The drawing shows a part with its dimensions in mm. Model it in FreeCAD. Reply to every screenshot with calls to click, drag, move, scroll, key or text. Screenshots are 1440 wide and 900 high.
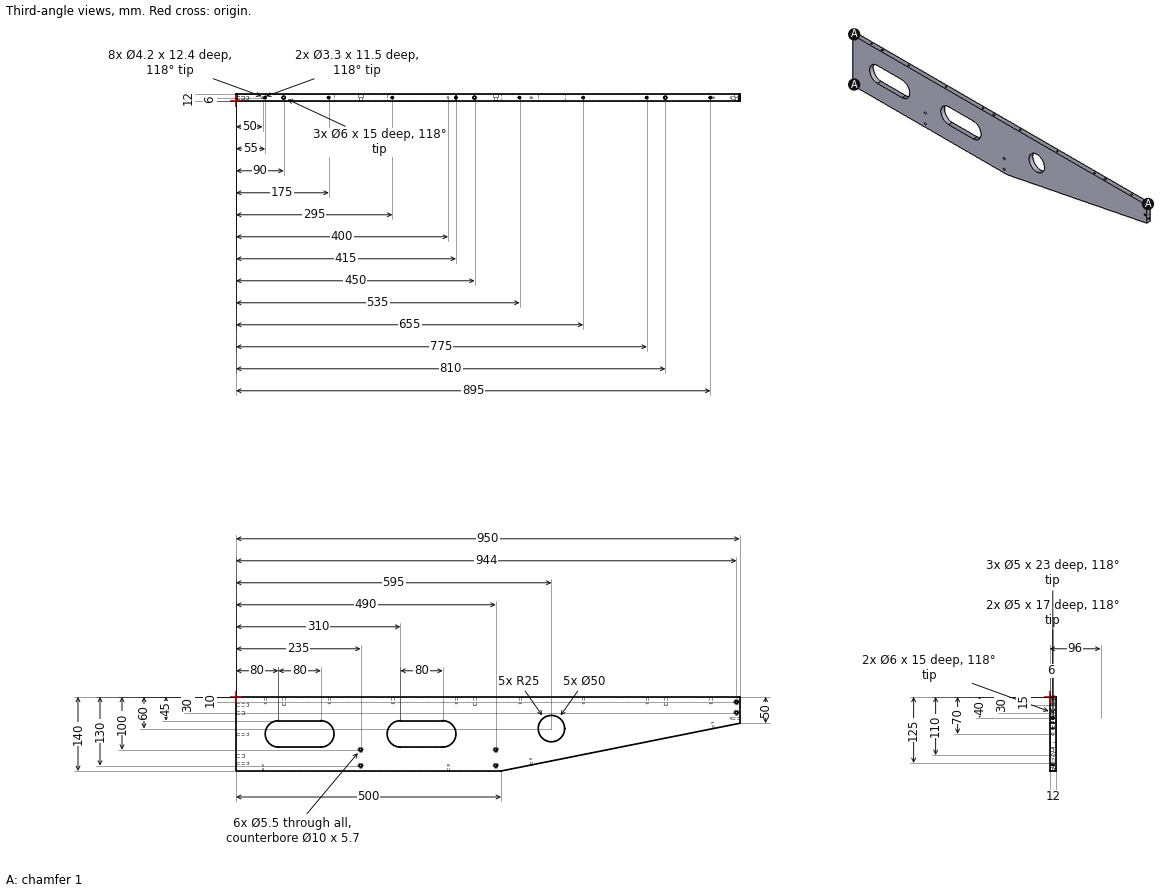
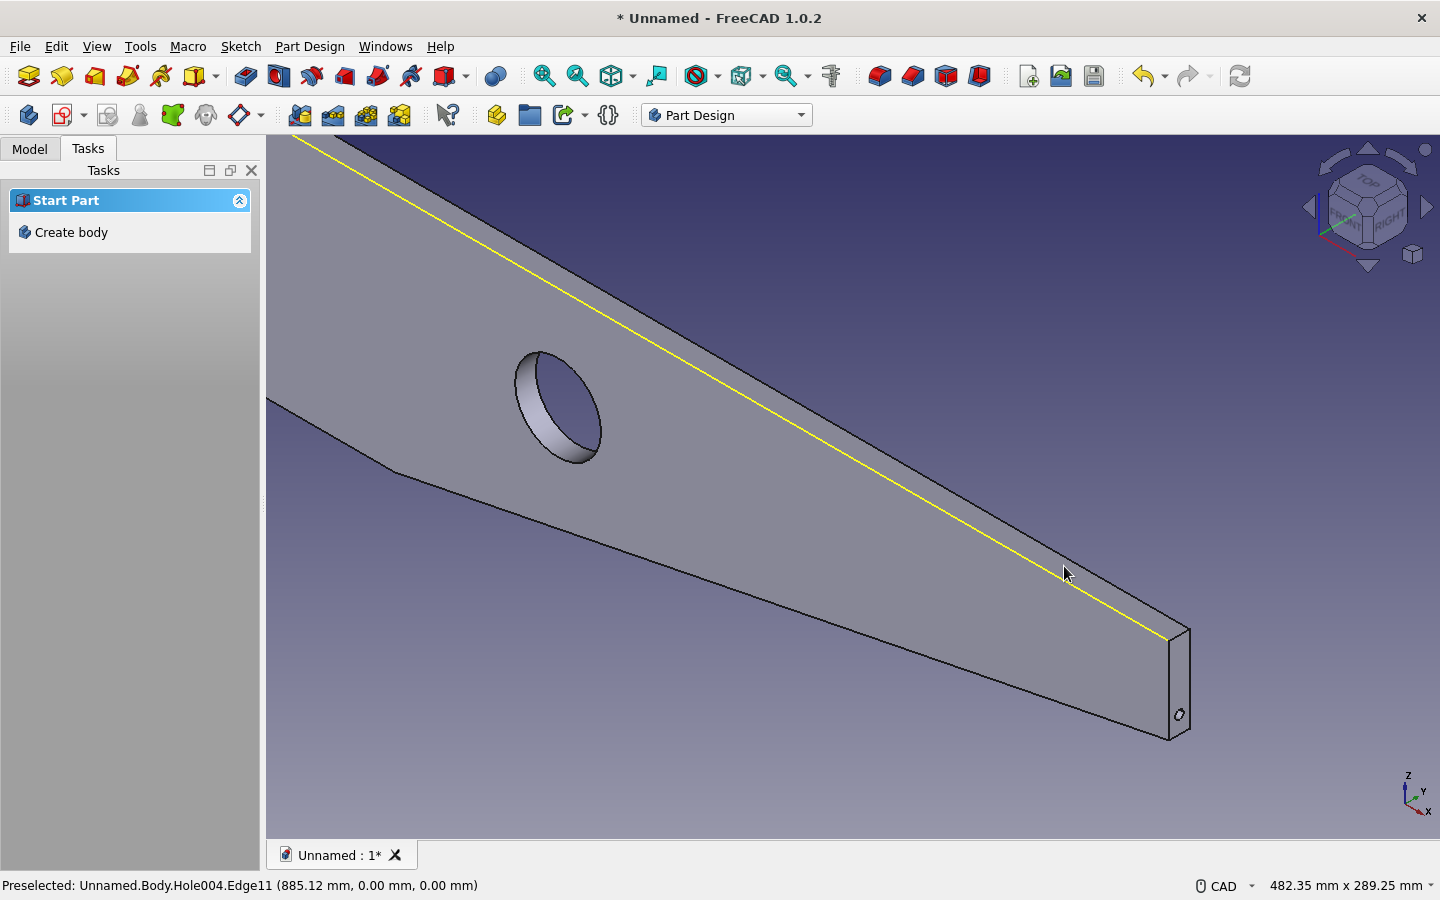
click(1063, 567)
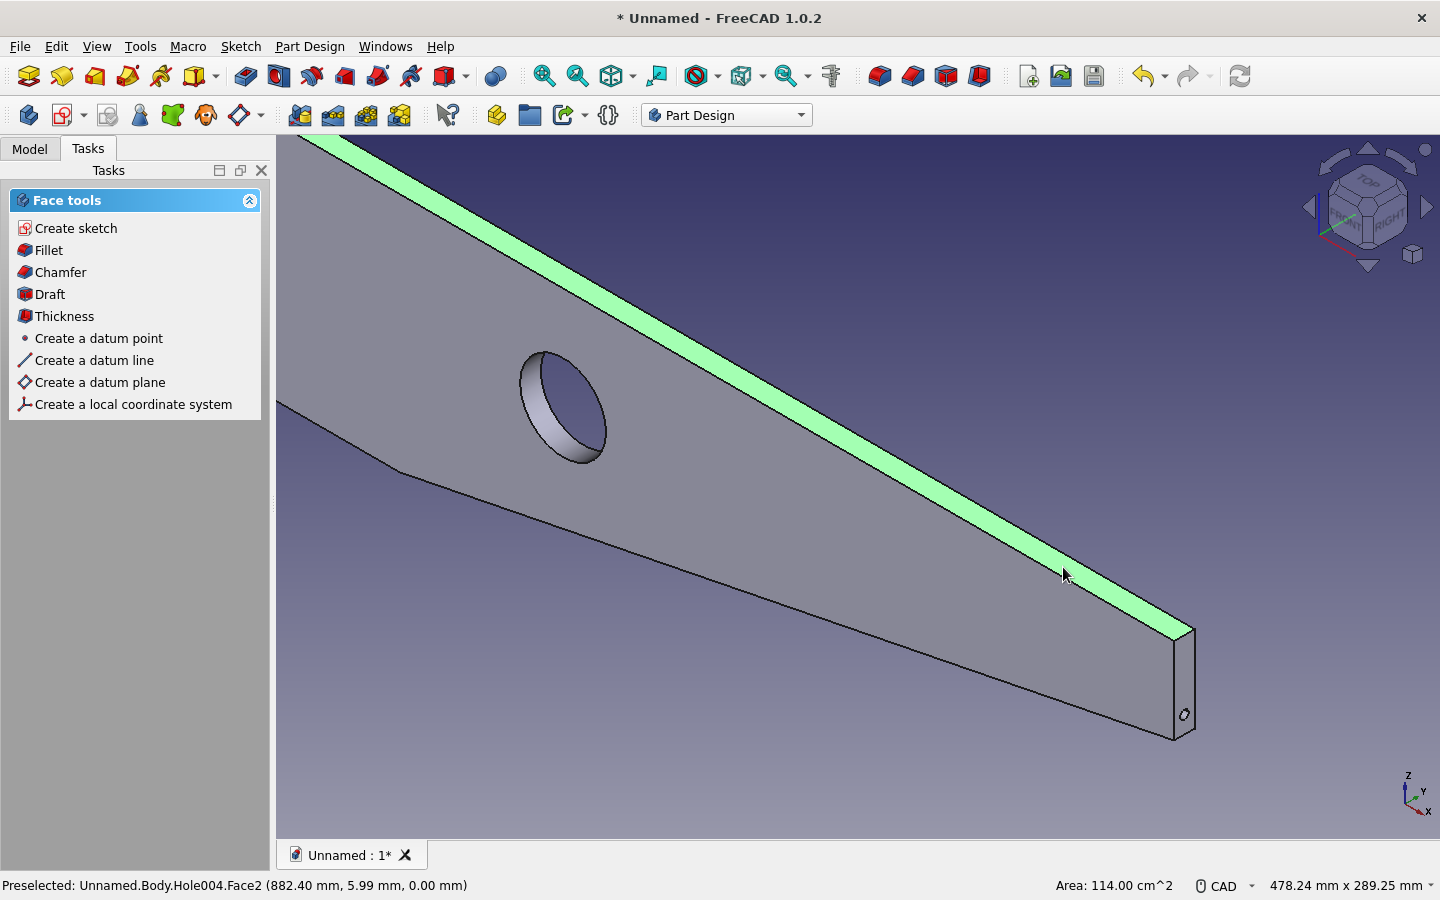
click(62, 116)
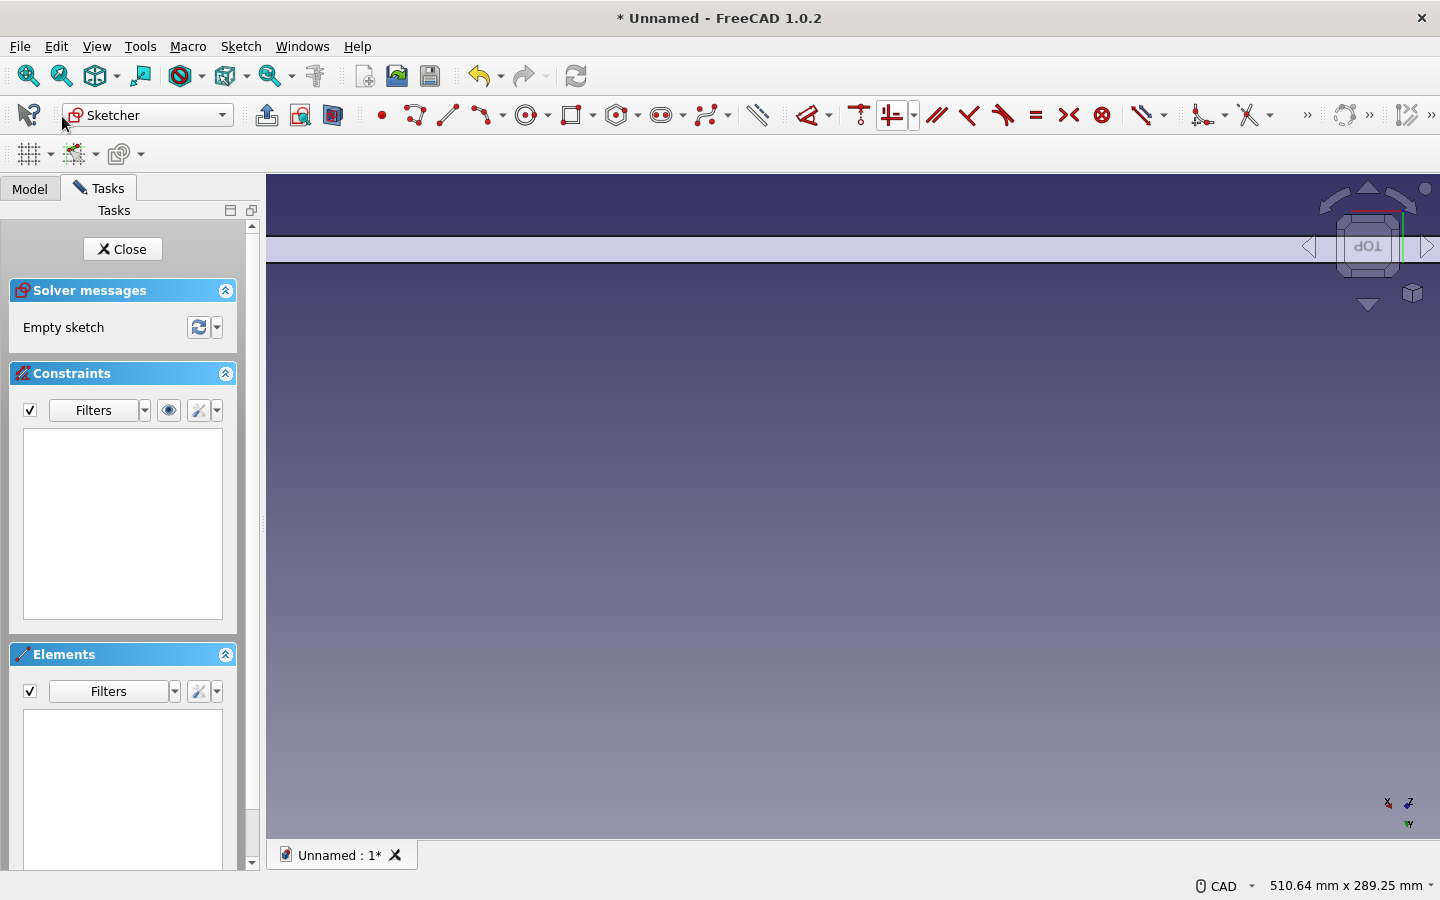
scroll(477, 659, down, 5)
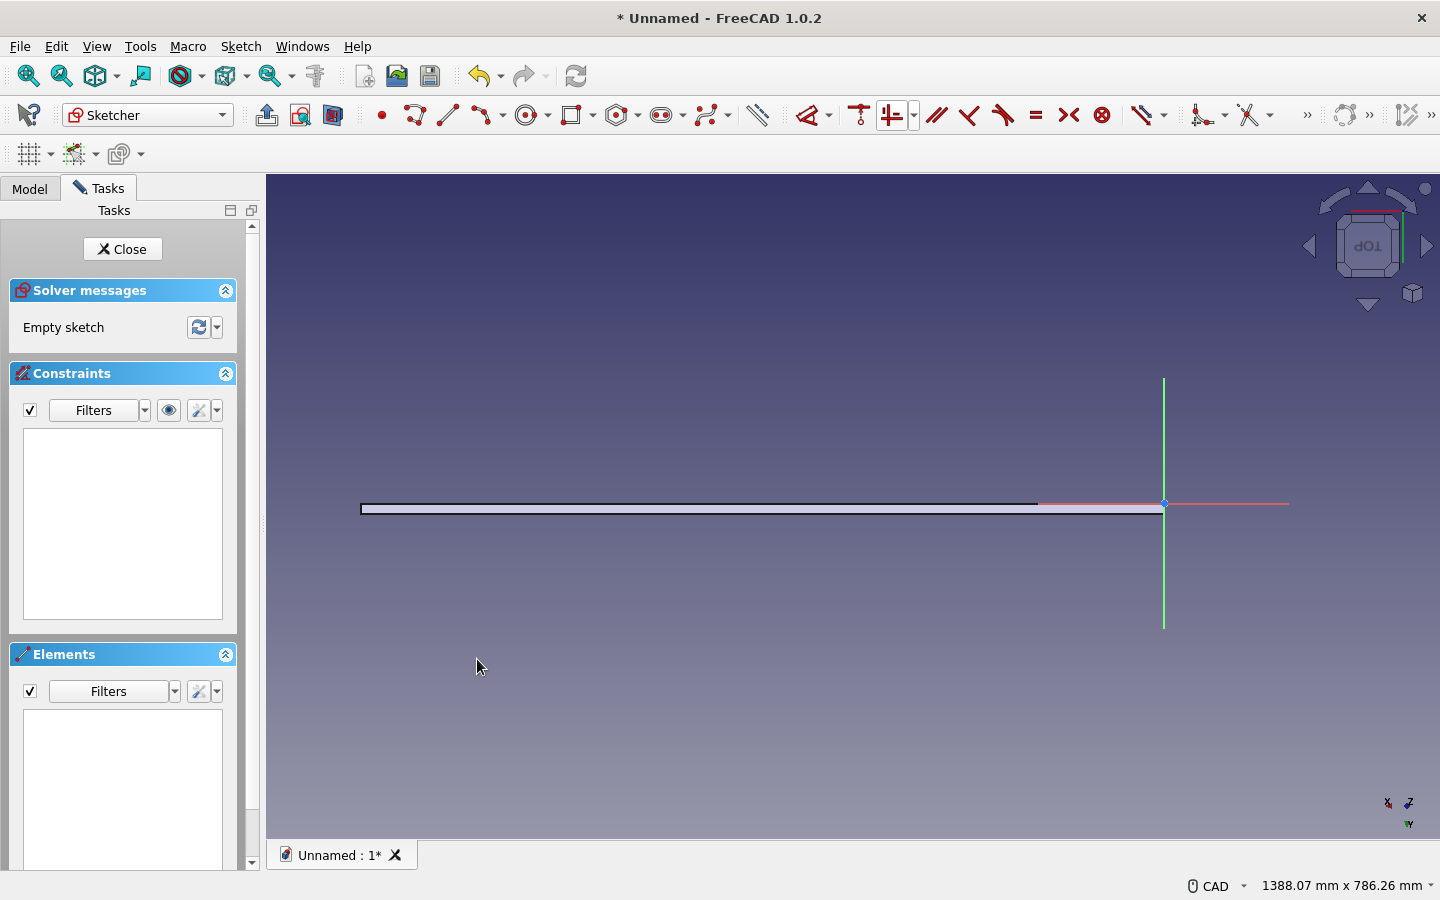
click(526, 116)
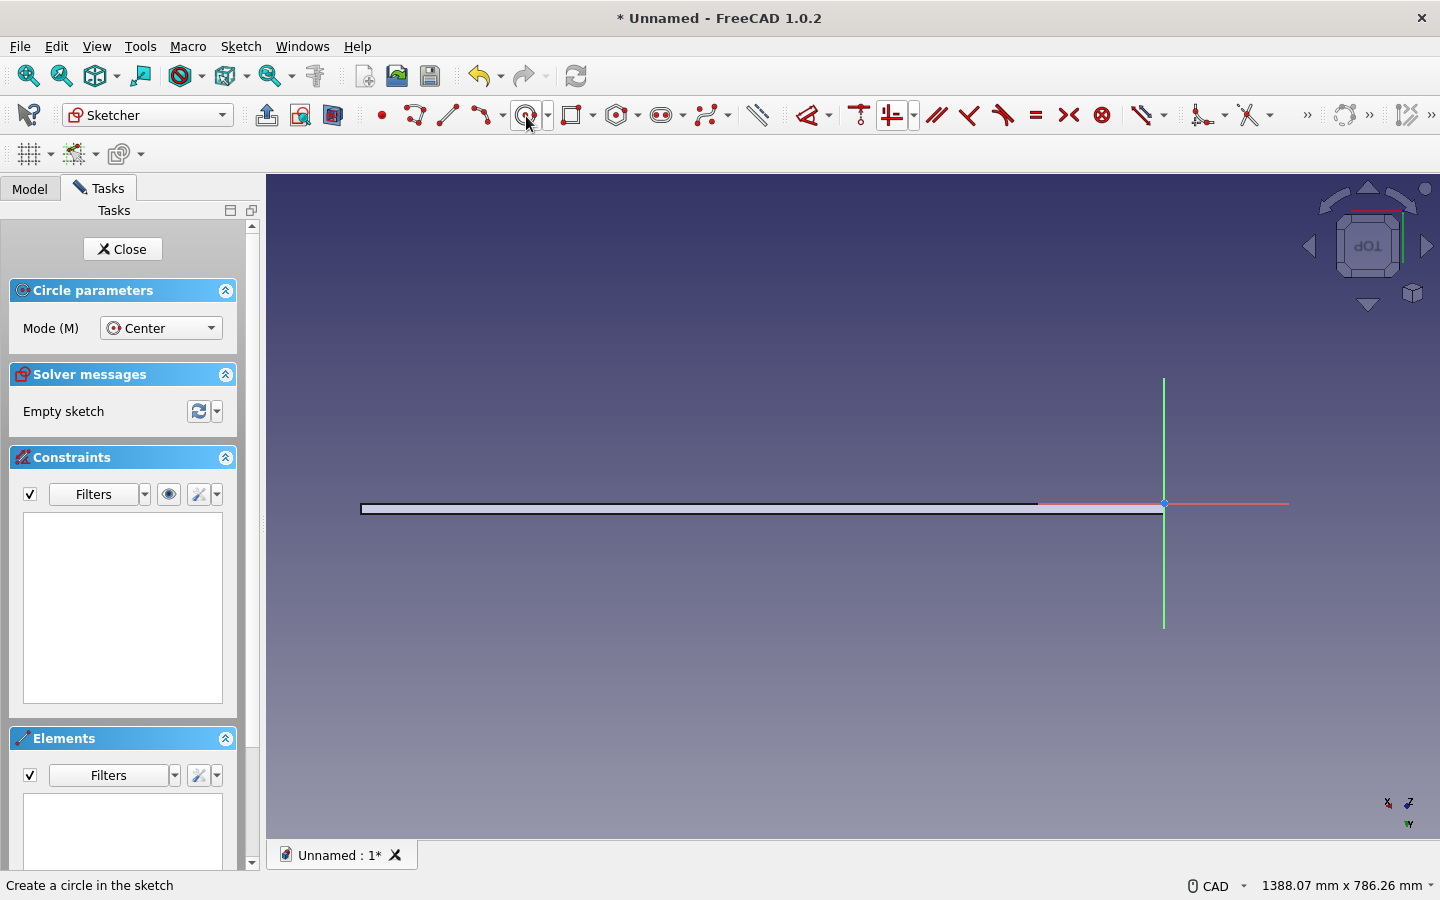
scroll(1118, 509, up, 13)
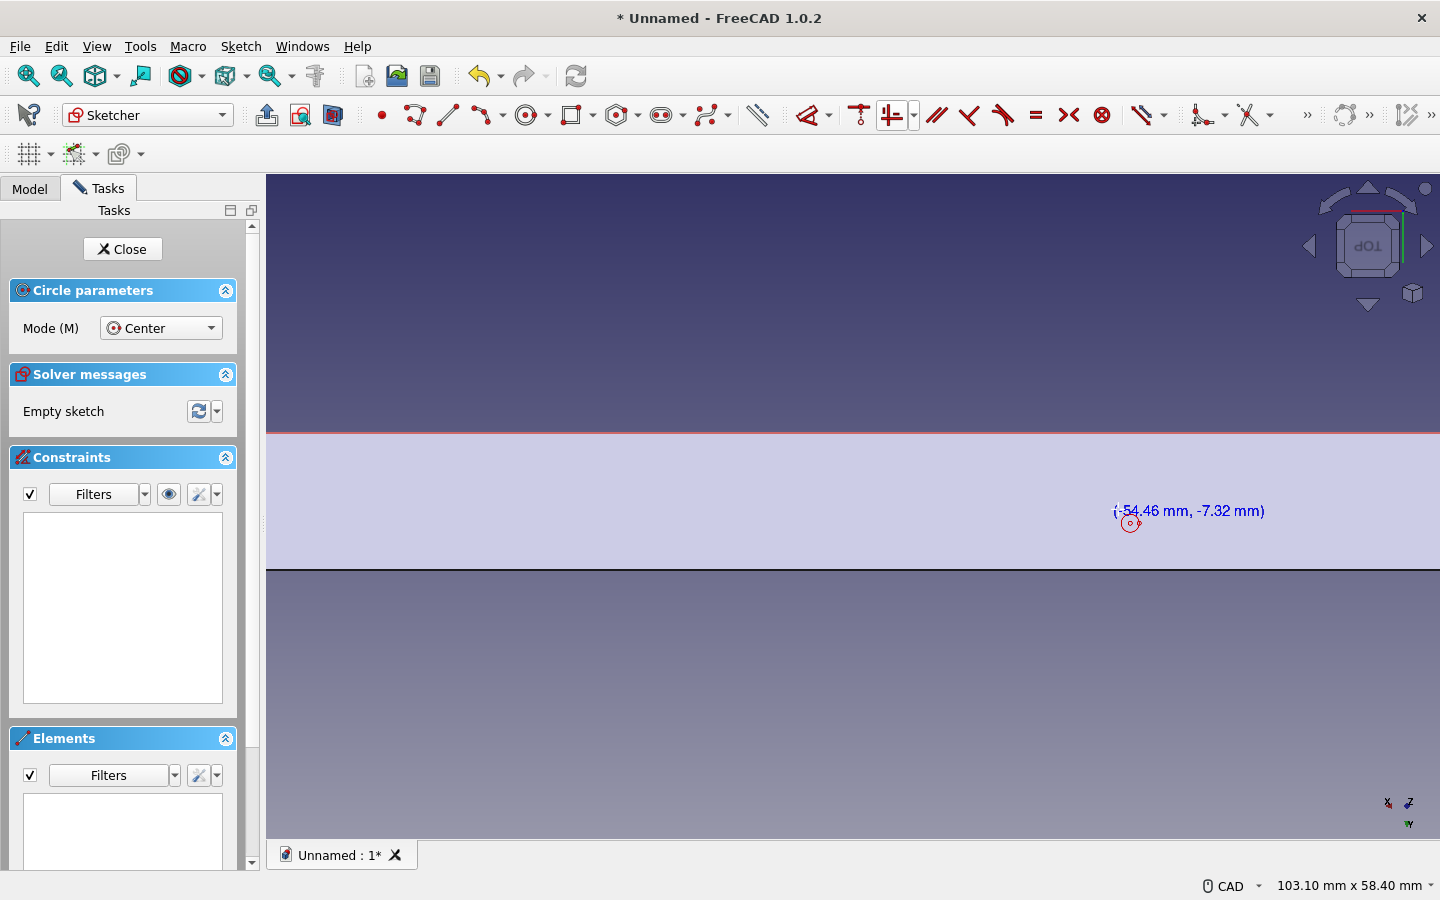
scroll(1119, 509, down, 13)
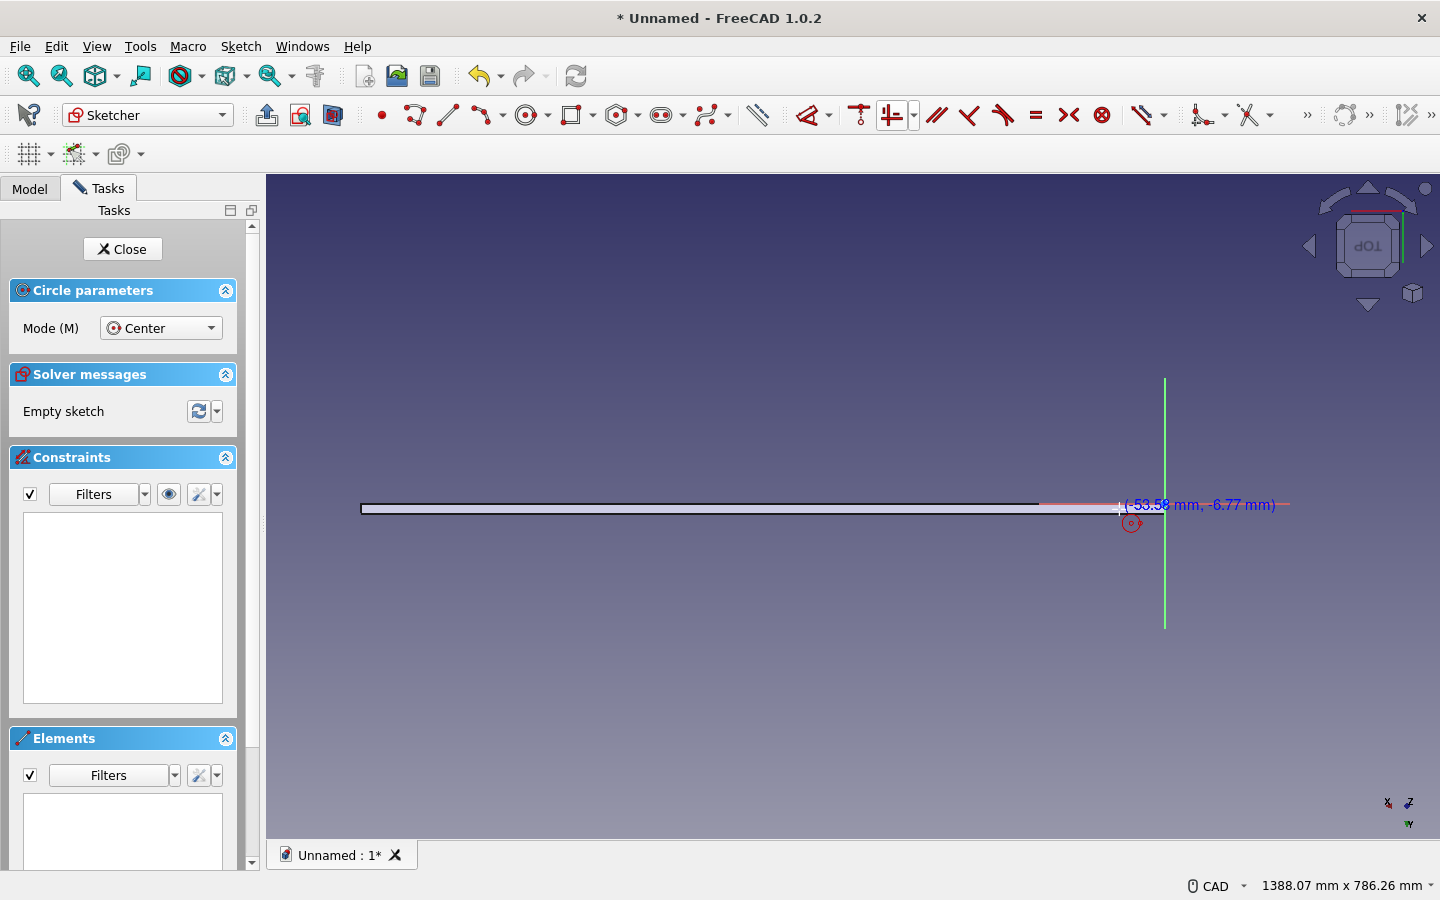
scroll(1118, 509, up, 6)